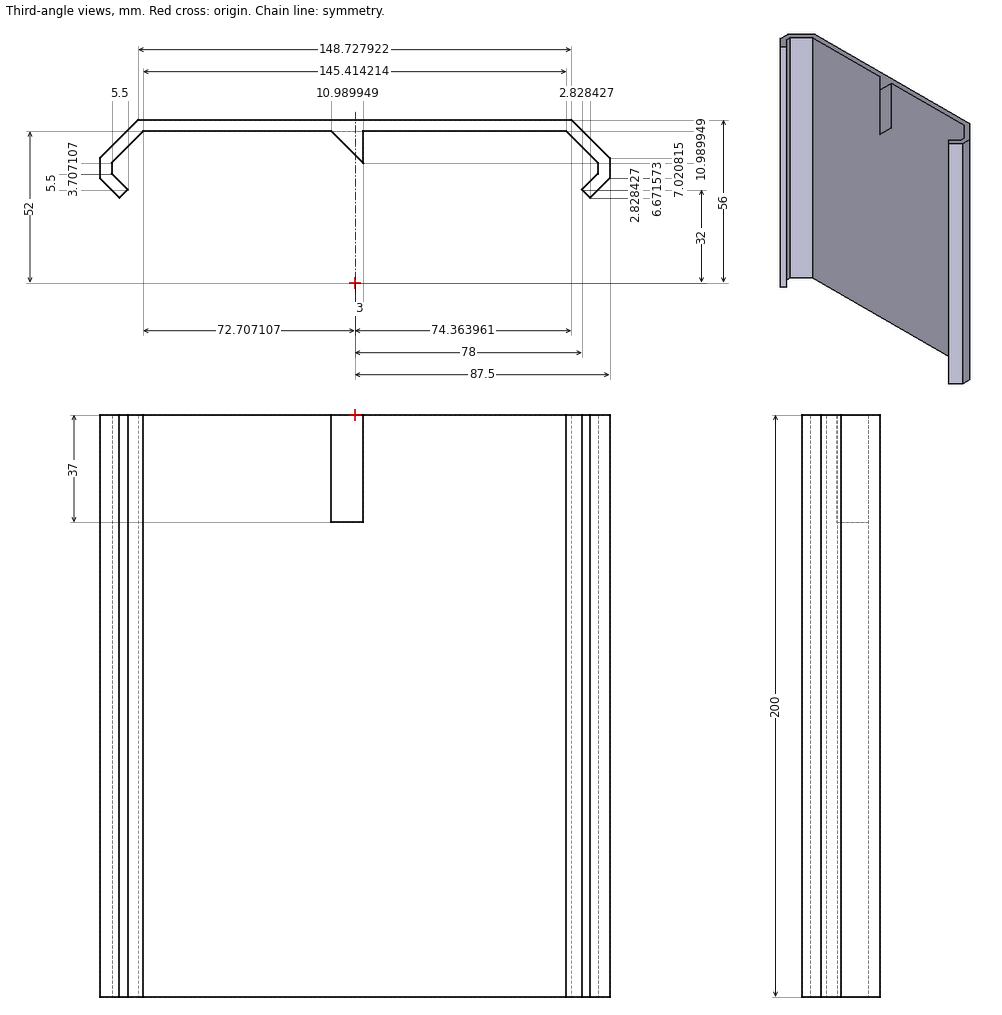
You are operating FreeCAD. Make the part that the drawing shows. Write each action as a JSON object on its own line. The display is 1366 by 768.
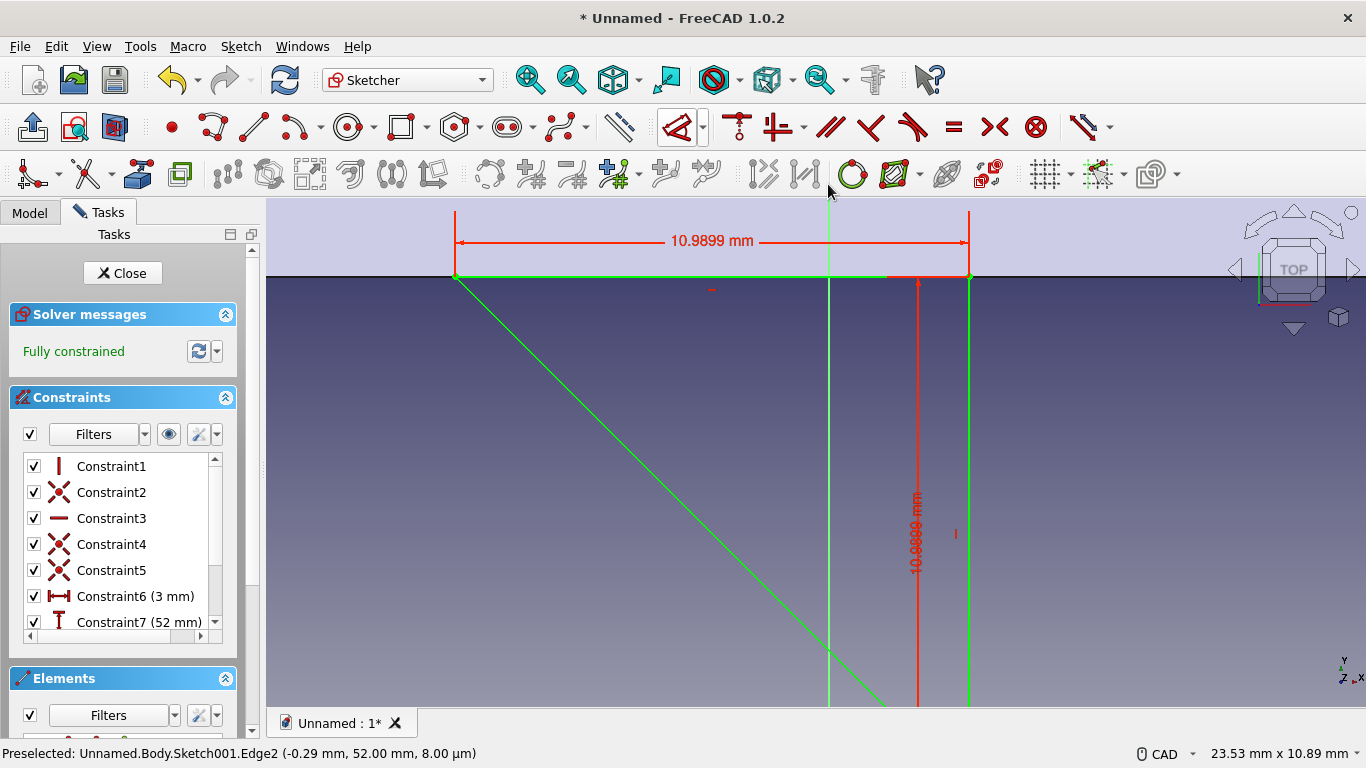
{"action": "left_click", "coordinate": [123, 273]}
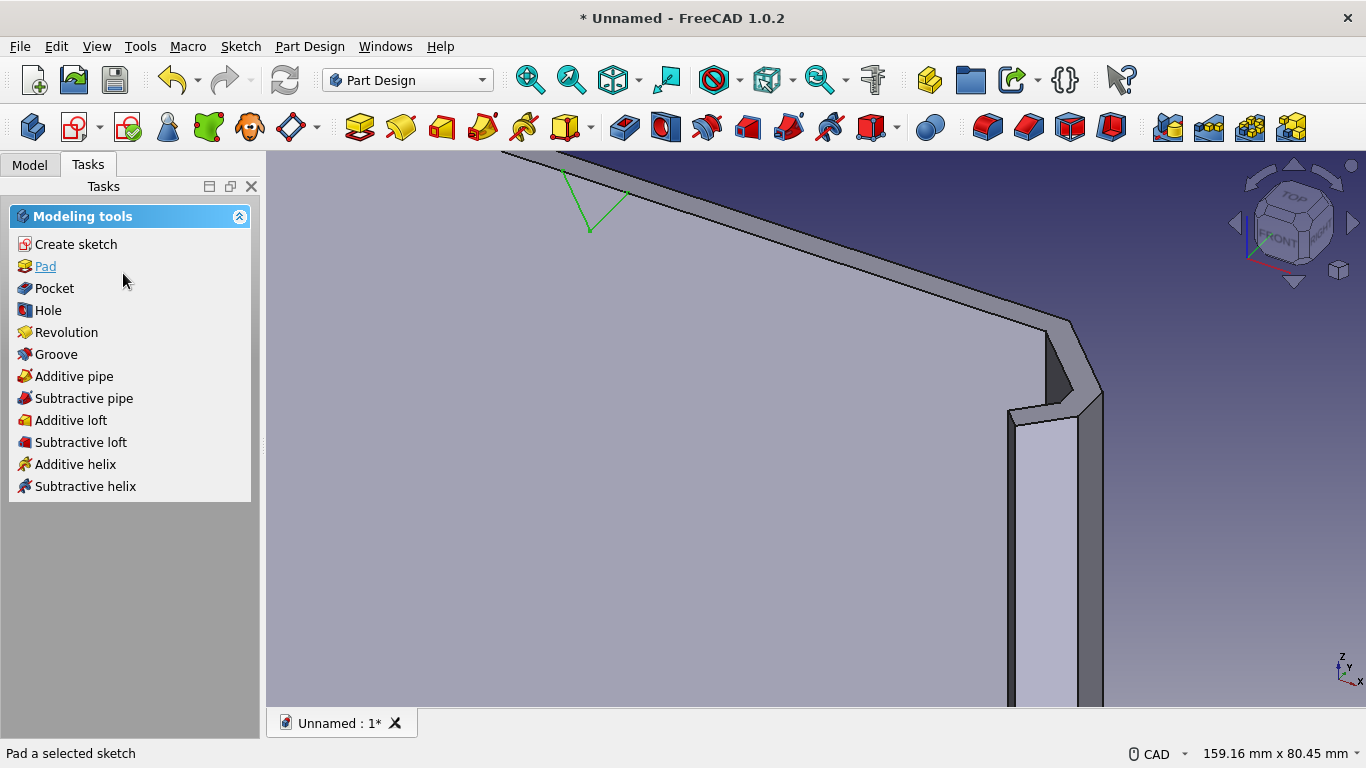
{"action": "left_click", "coordinate": [360, 128]}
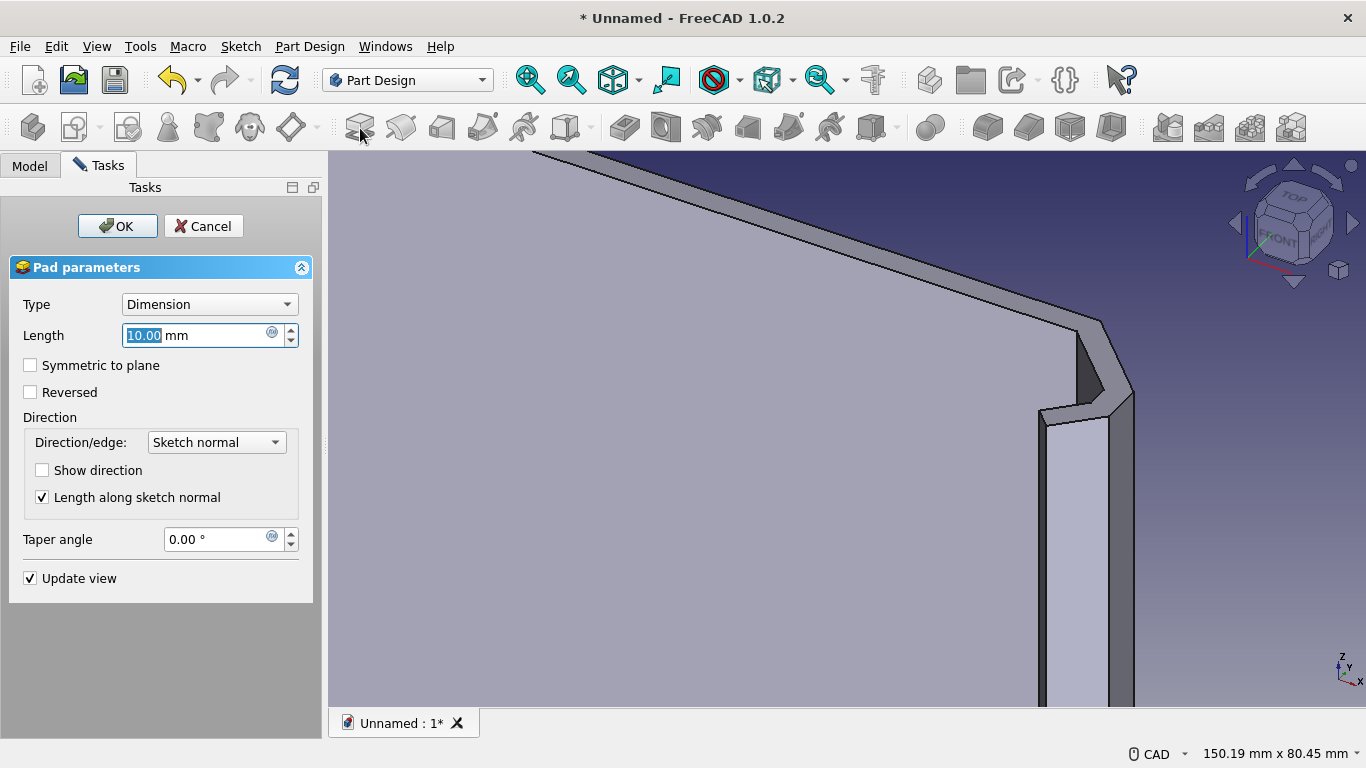
{"action": "type", "text": "37"}
{"action": "key", "text": "Tab"}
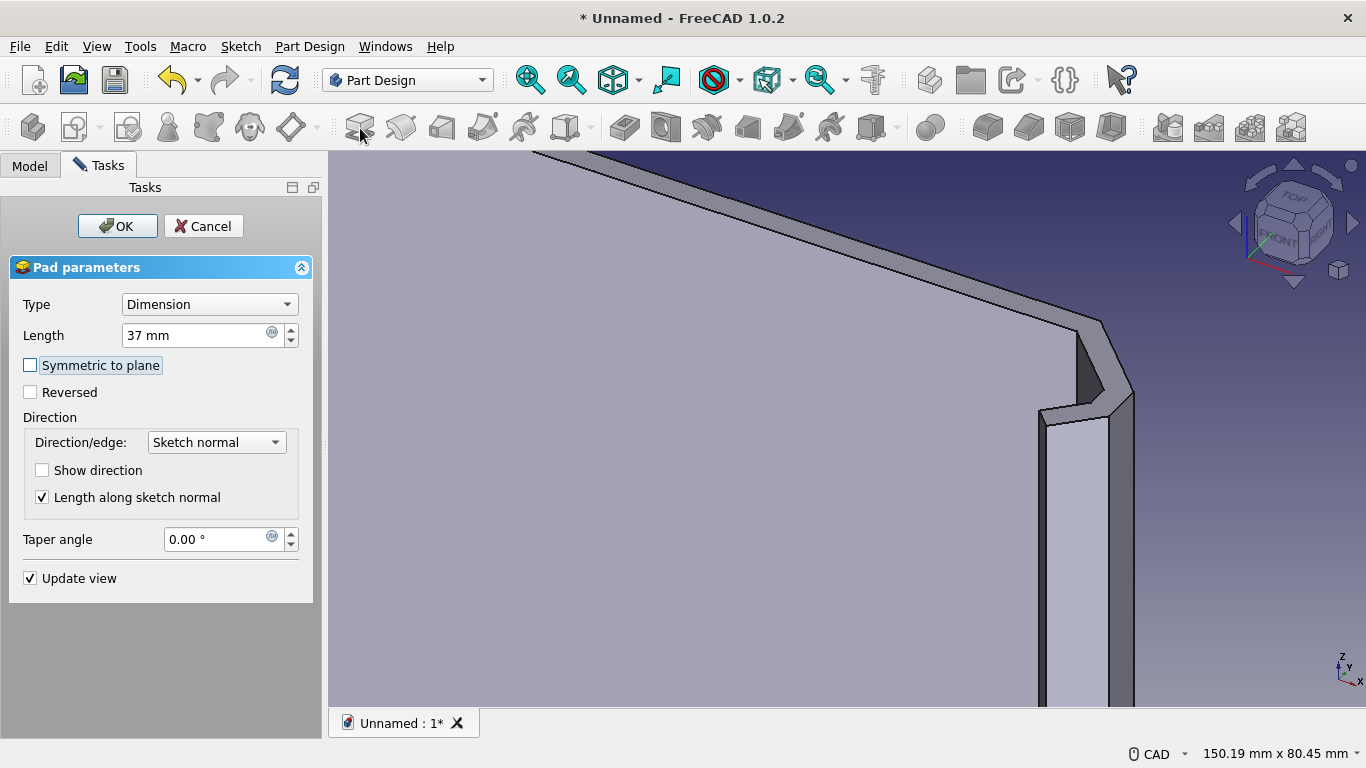
{"action": "left_click", "coordinate": [31, 392]}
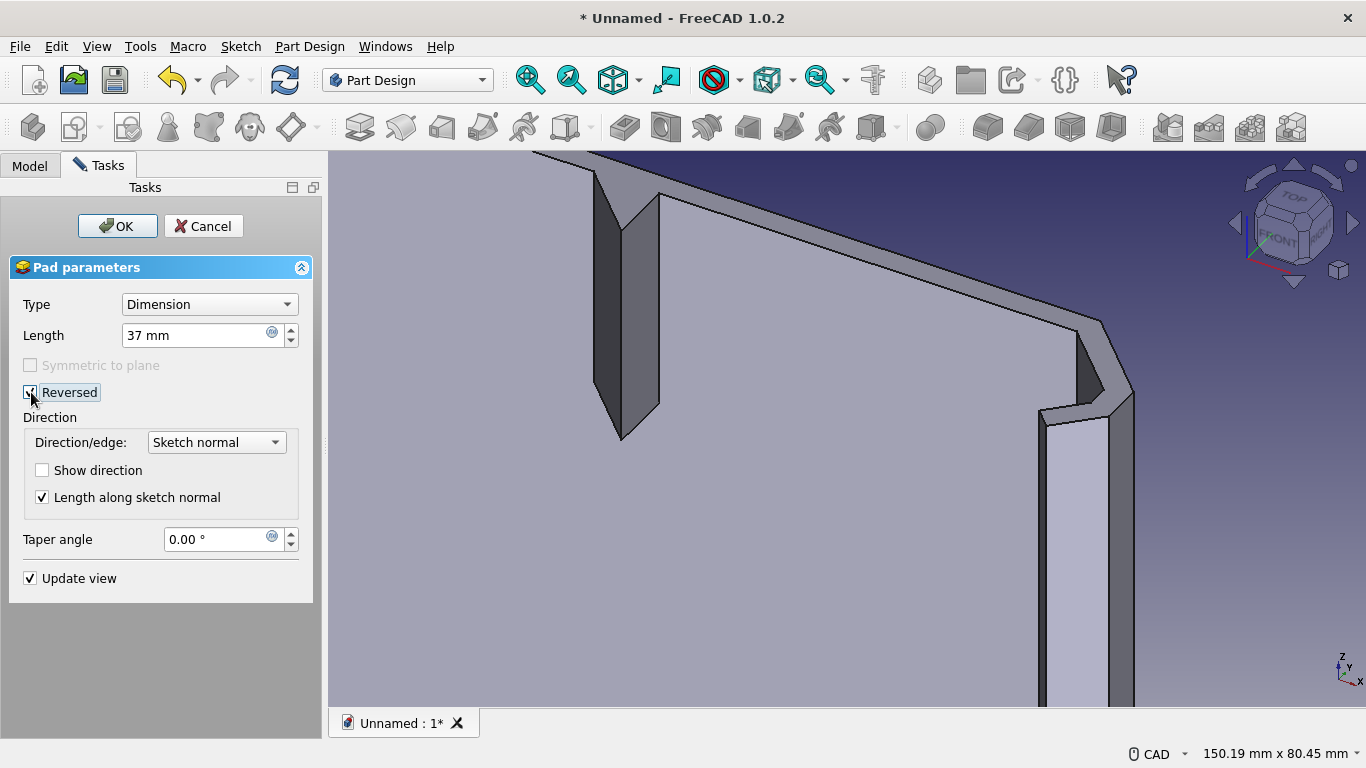
{"action": "left_click", "coordinate": [118, 226]}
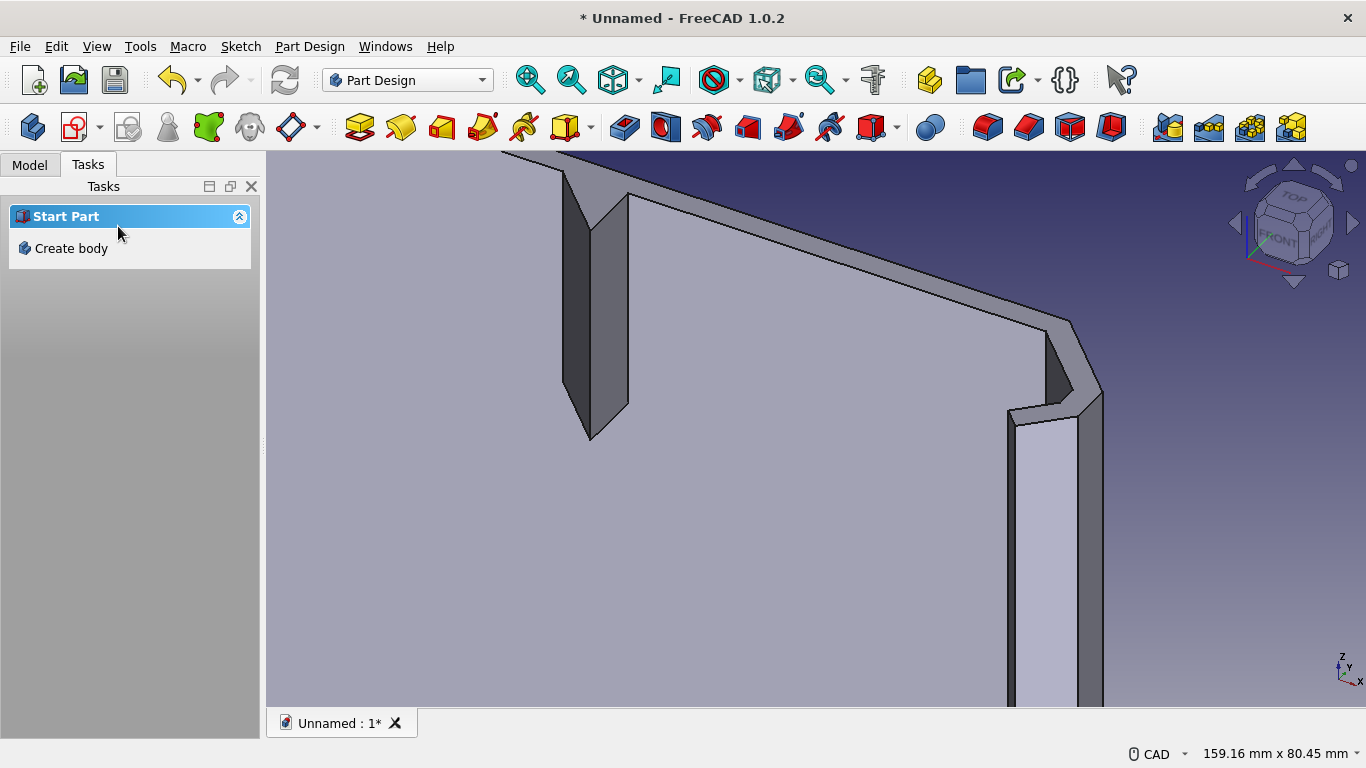
{"action": "key", "text": "0"}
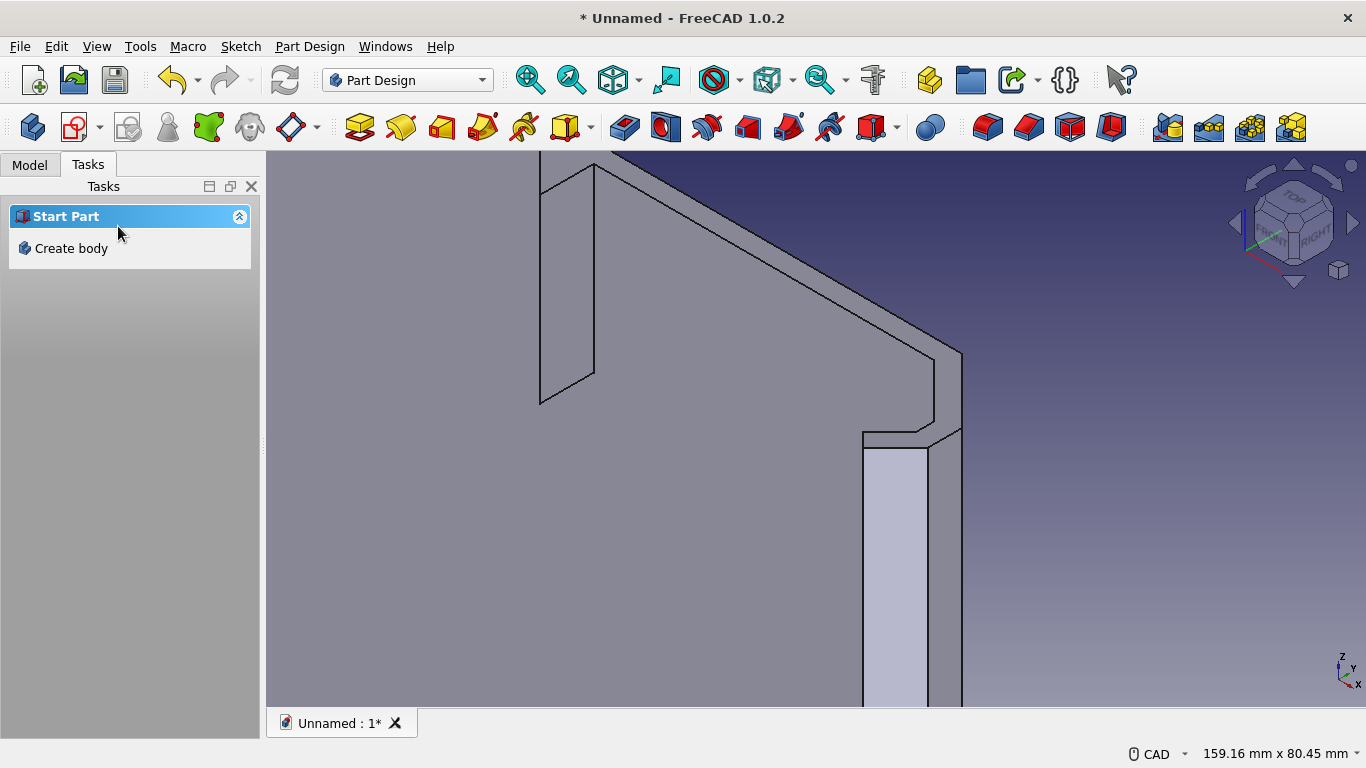
{"action": "left_click", "coordinate": [531, 80]}